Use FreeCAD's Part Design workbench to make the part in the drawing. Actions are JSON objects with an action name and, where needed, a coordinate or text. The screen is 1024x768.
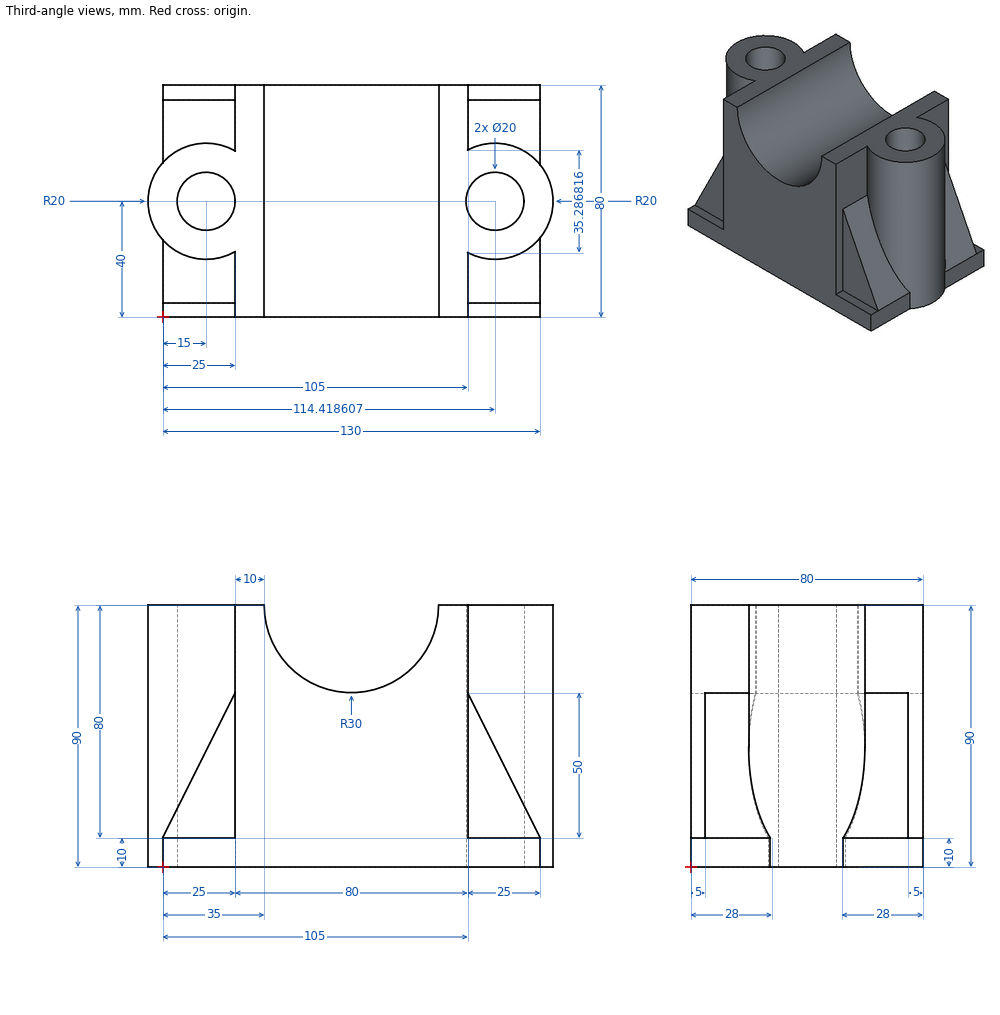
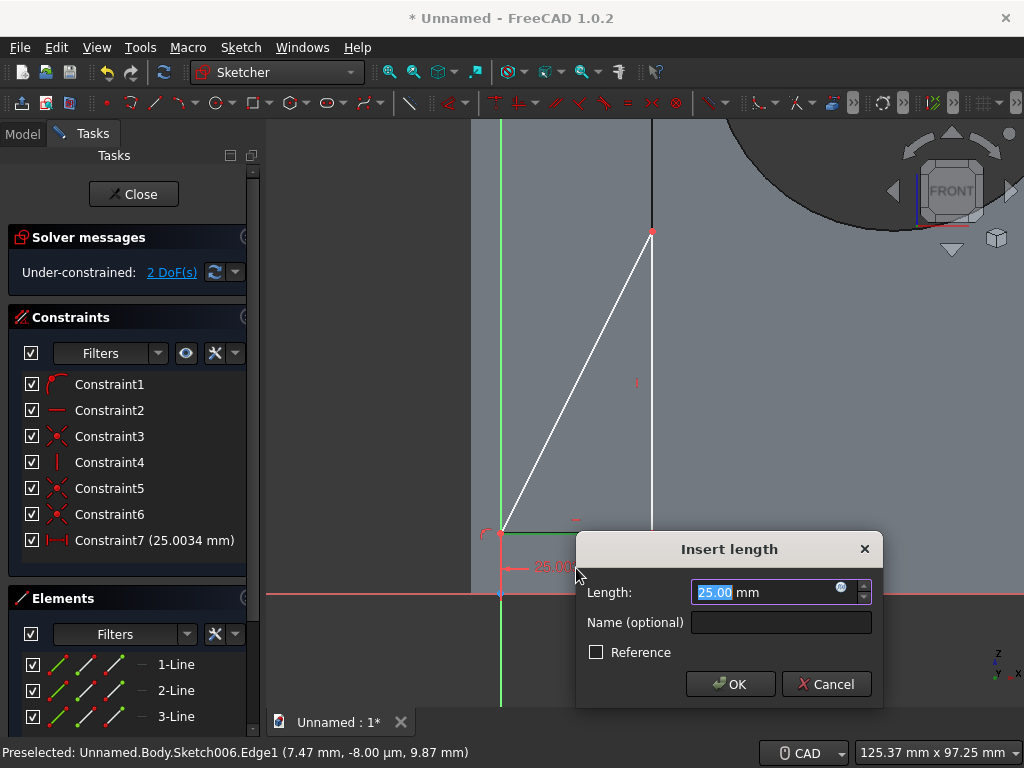
{"action": "type", "text": "25"}
{"action": "key", "text": "Return"}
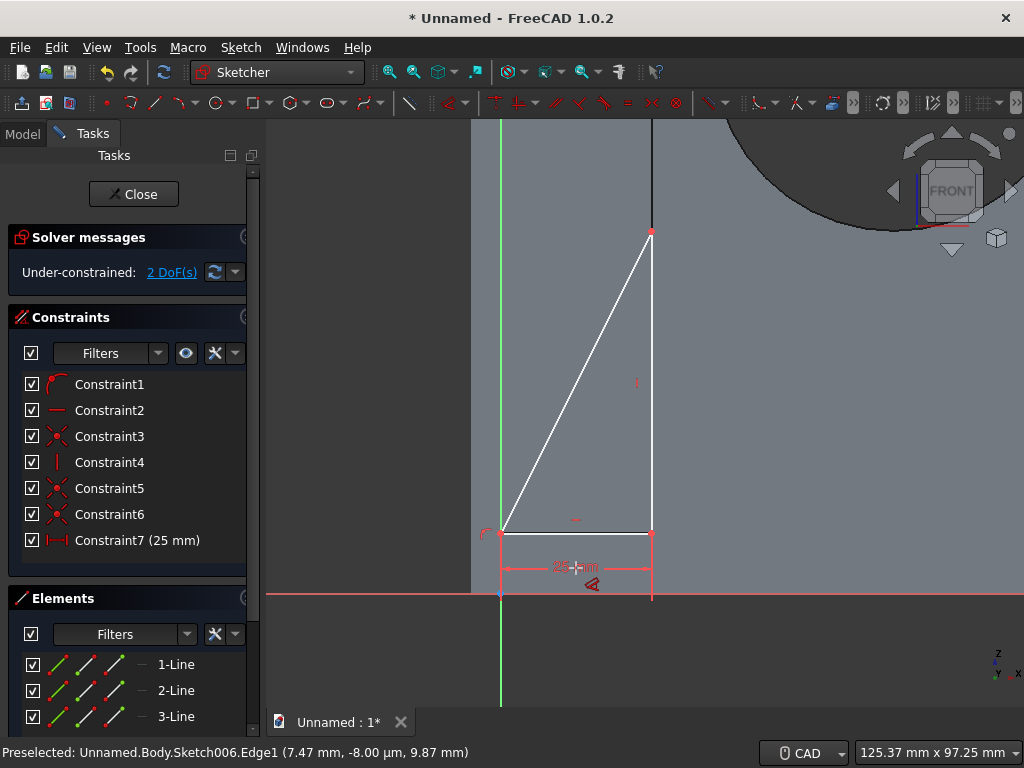
{"action": "left_click", "coordinate": [652, 443]}
{"action": "left_click", "coordinate": [686, 383]}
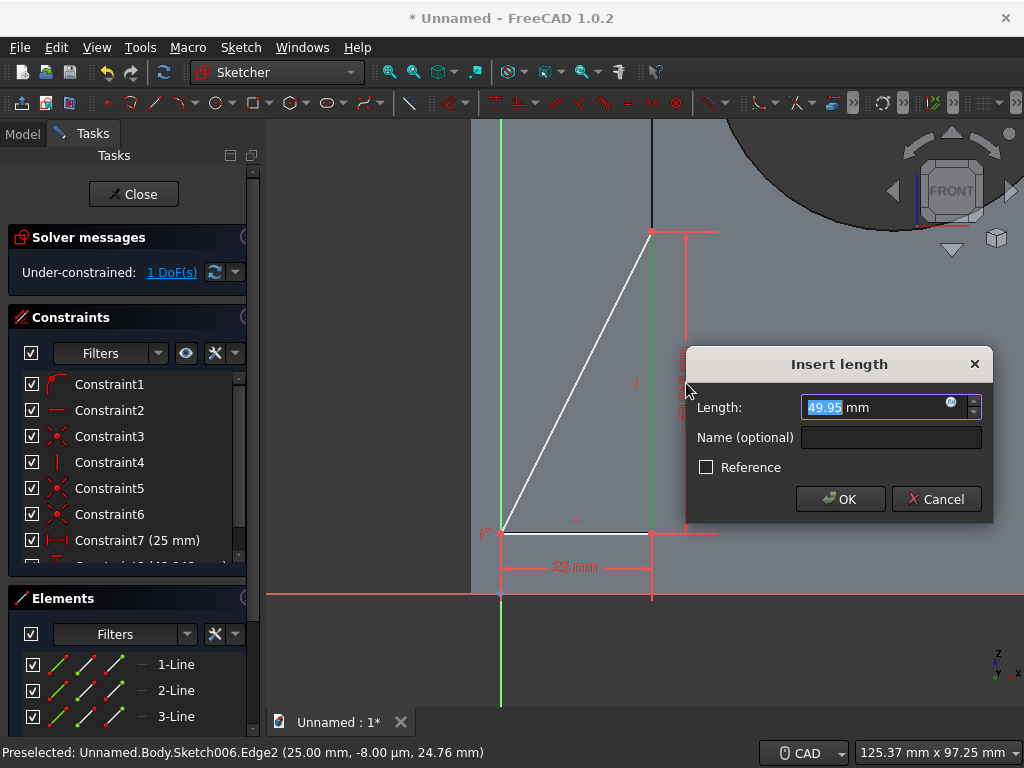
{"action": "type", "text": "50"}
{"action": "key", "text": "Return"}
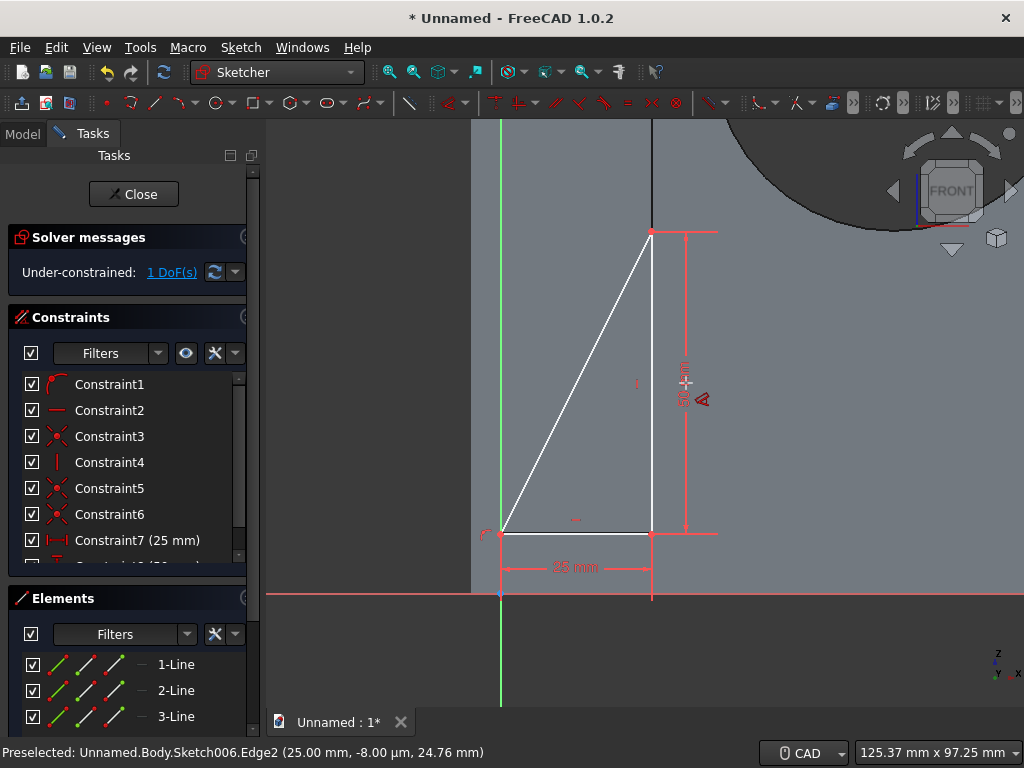
{"action": "left_click", "coordinate": [501, 534]}
{"action": "left_click", "coordinate": [467, 564]}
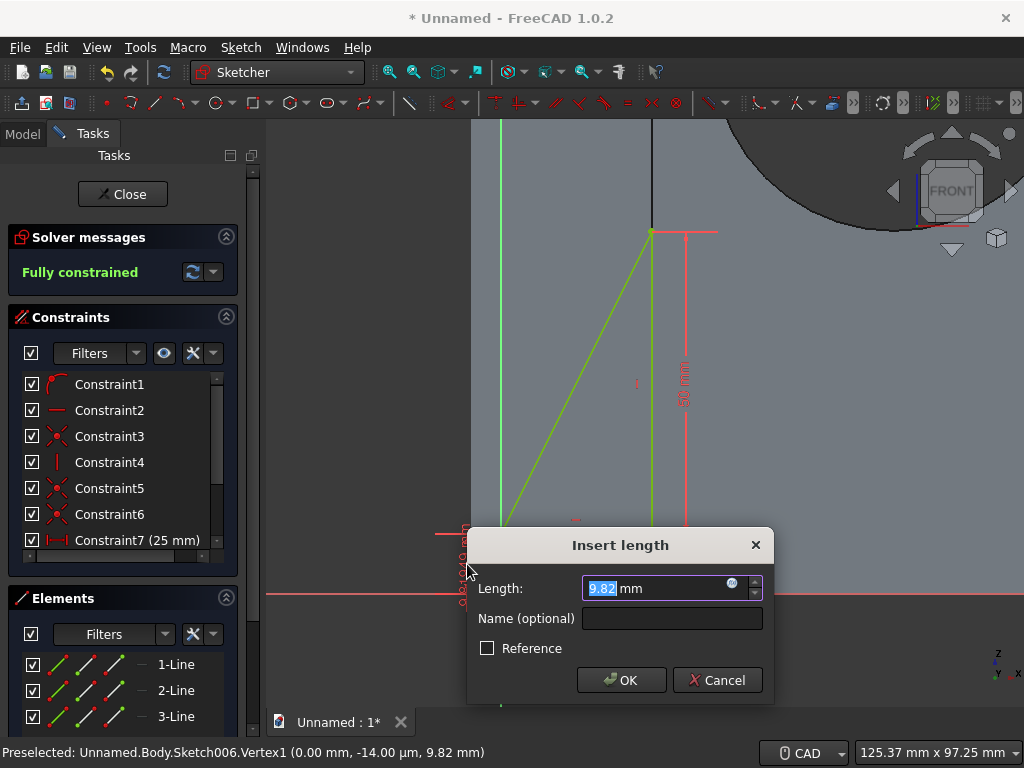
{"action": "type", "text": "10"}
{"action": "key", "text": "Return"}
{"action": "key", "text": "Escape"}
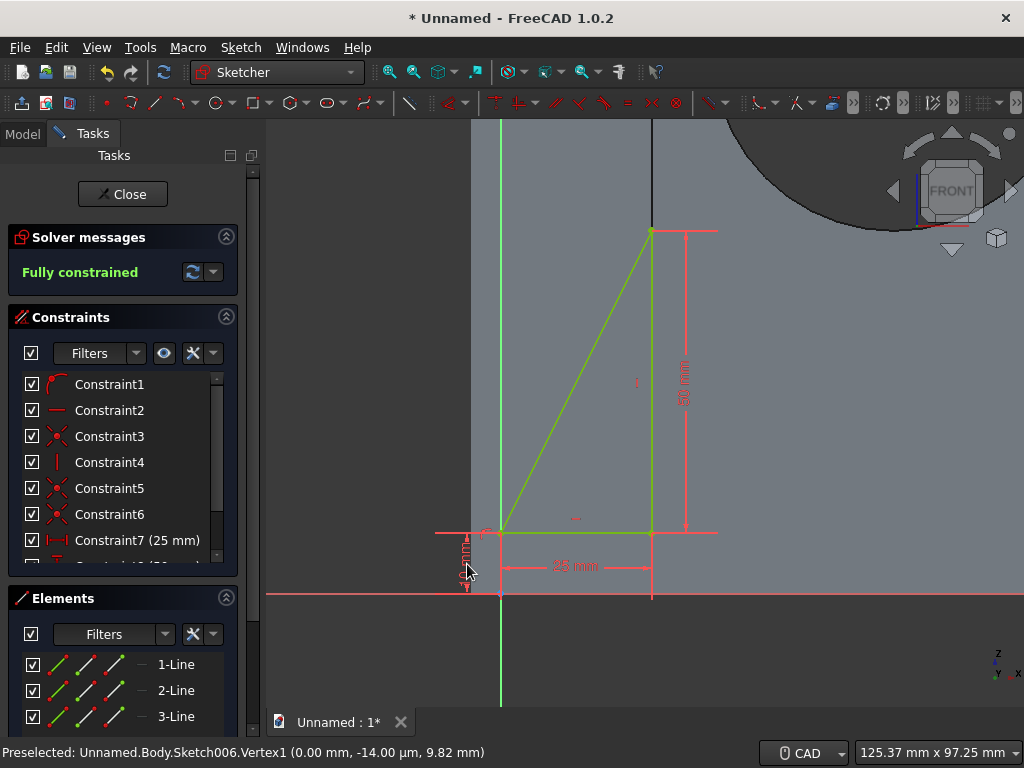
{"action": "left_click", "coordinate": [123, 194]}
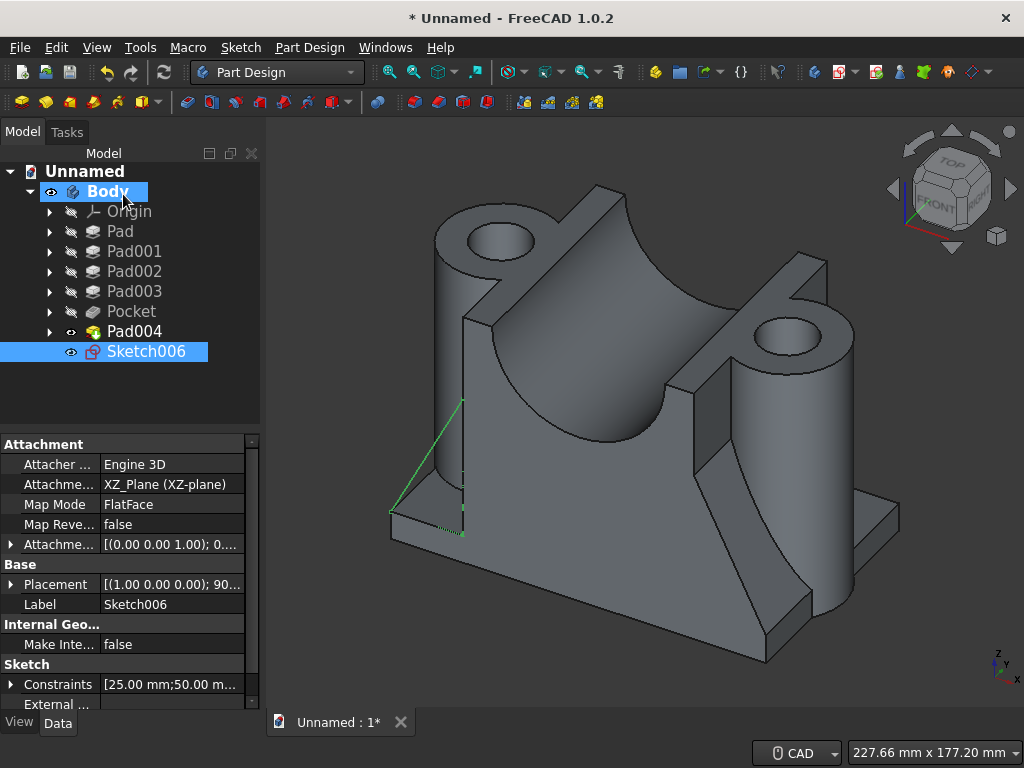
{"action": "left_click", "coordinate": [22, 102]}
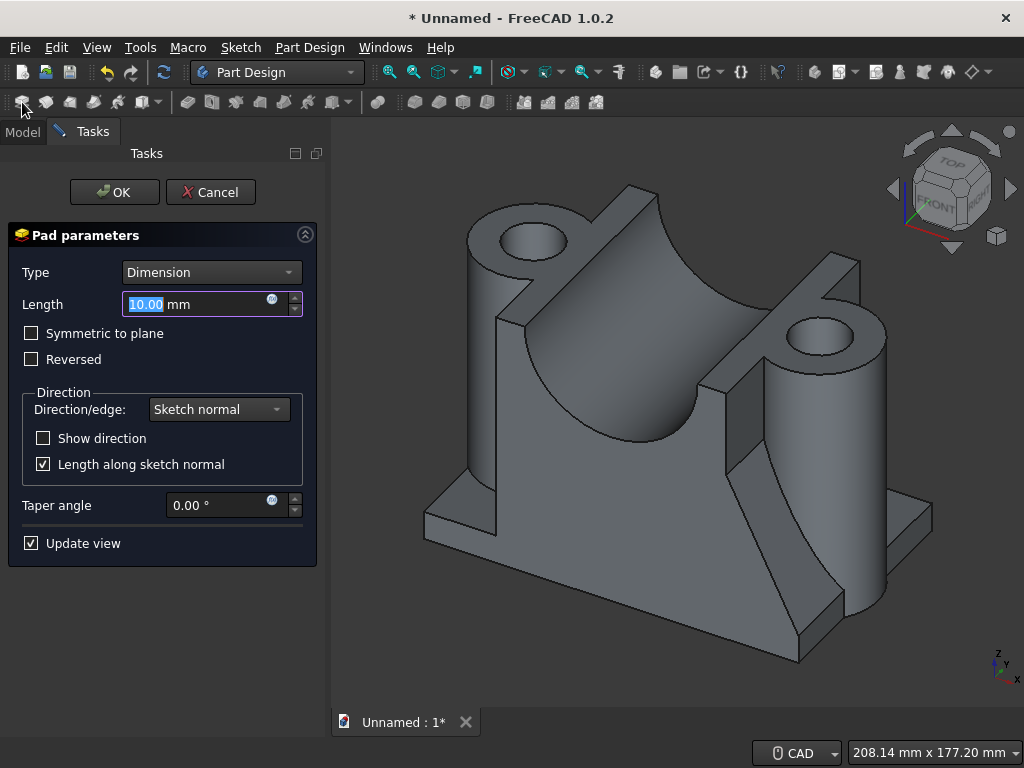
{"action": "type", "text": "28"}
{"action": "key", "text": "Tab"}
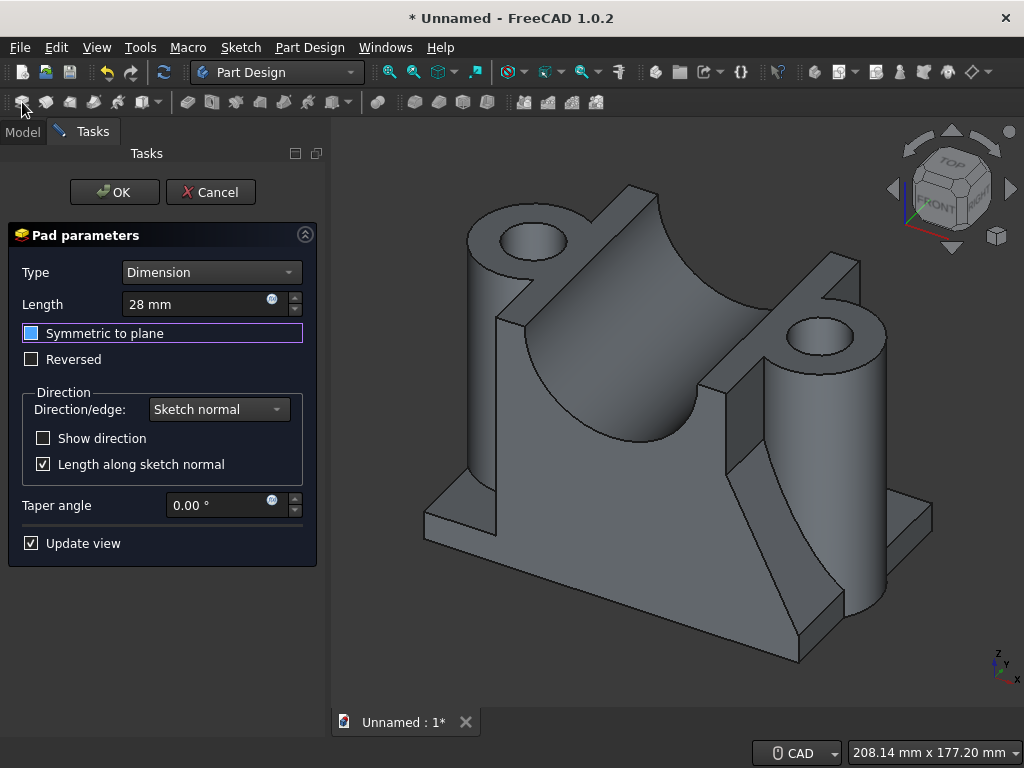
{"action": "left_click", "coordinate": [30, 359]}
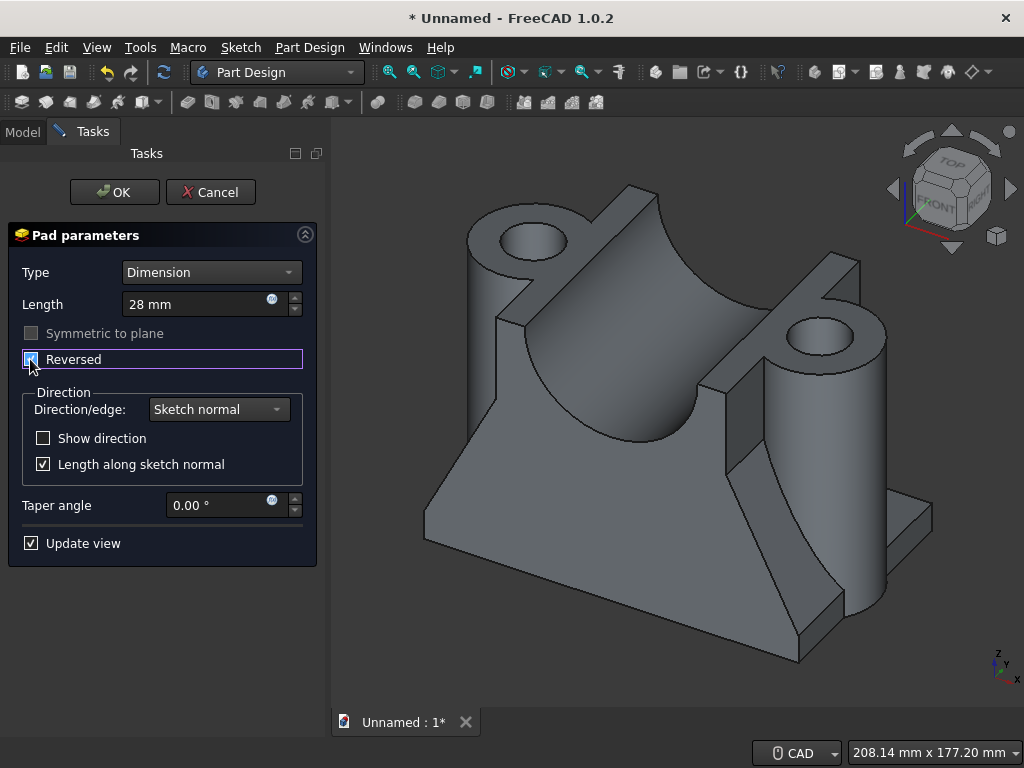
{"action": "left_click", "coordinate": [115, 192]}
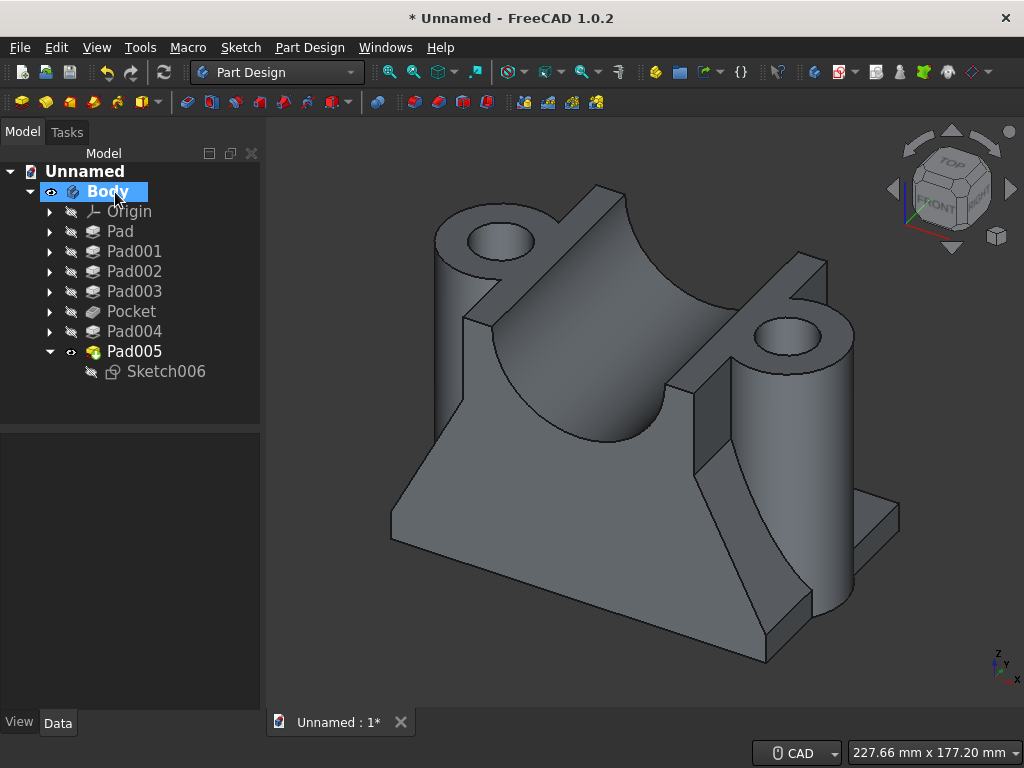
{"action": "key", "text": "4"}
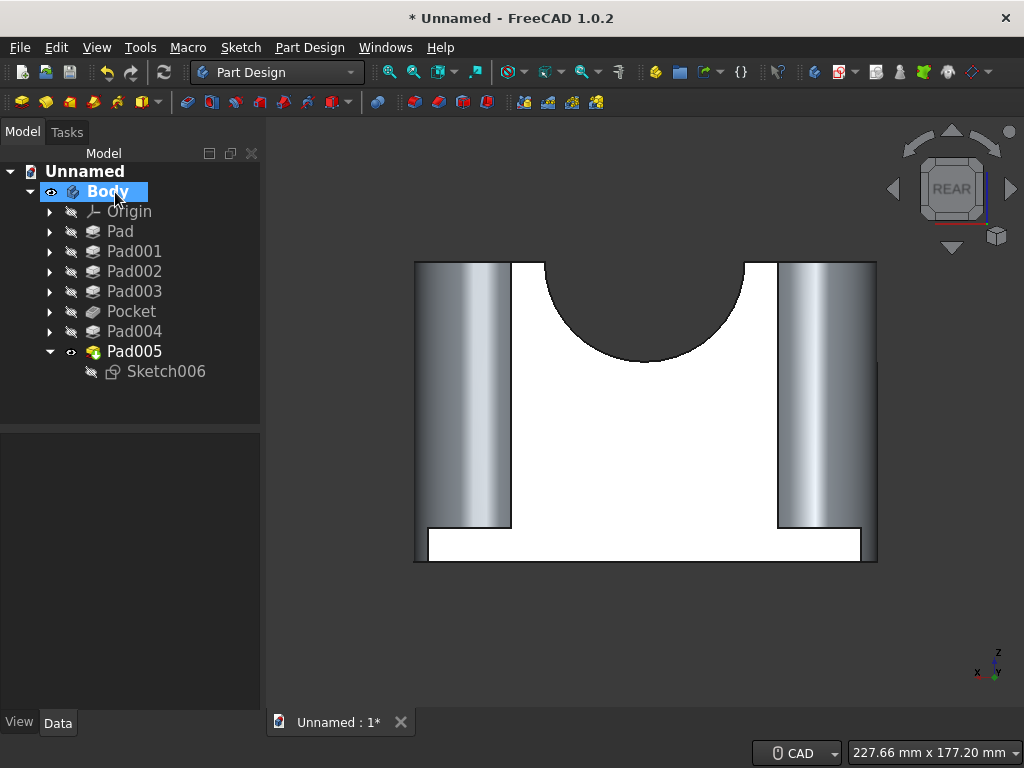
{"action": "left_click", "coordinate": [645, 454]}